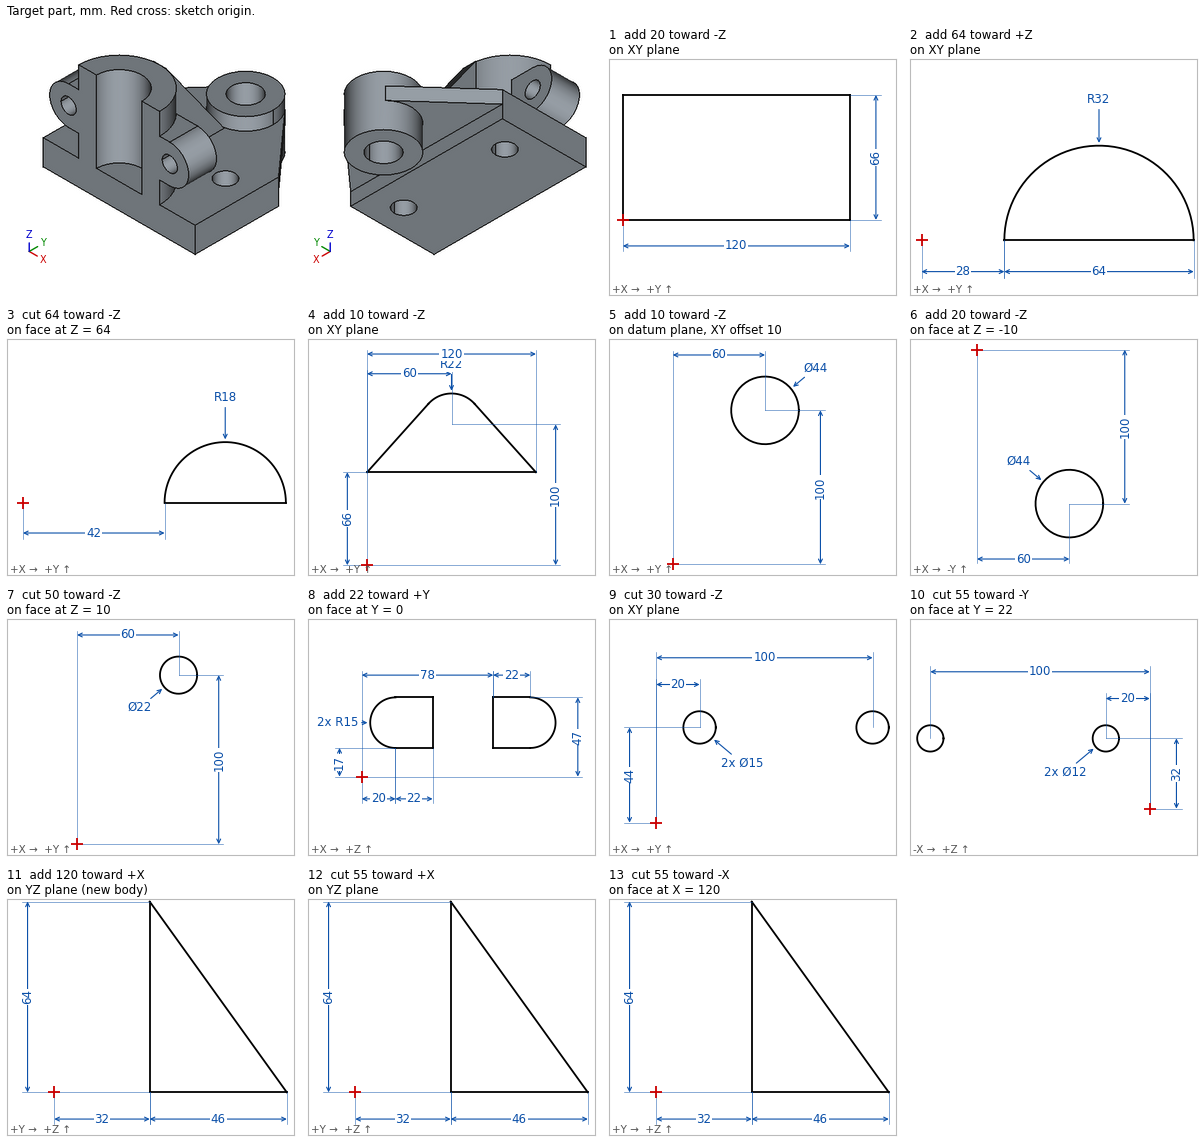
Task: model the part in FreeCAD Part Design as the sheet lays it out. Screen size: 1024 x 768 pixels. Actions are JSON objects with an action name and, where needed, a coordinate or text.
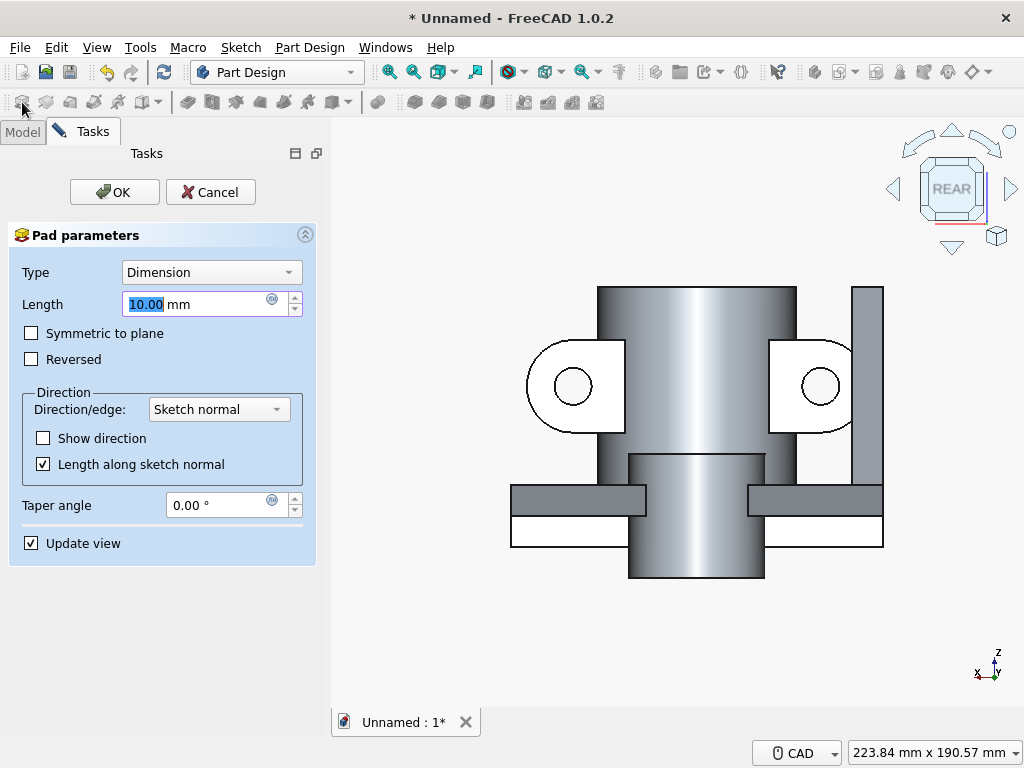
{"action": "type", "text": "120"}
{"action": "key", "text": "Tab"}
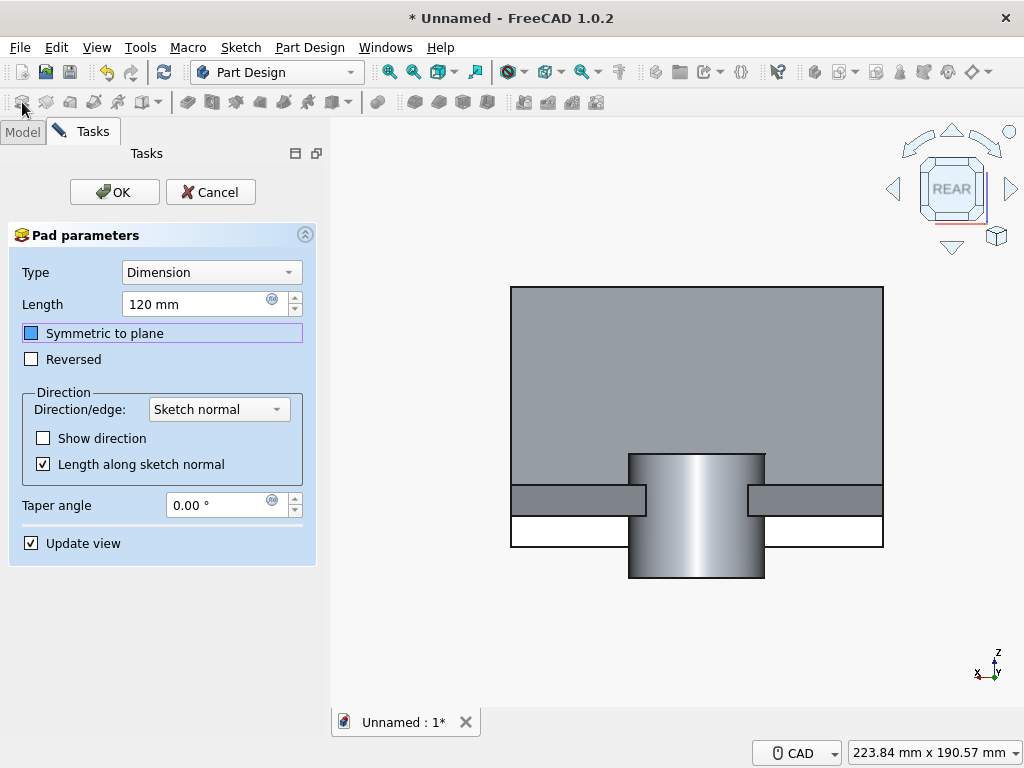
{"action": "left_click", "coordinate": [115, 192]}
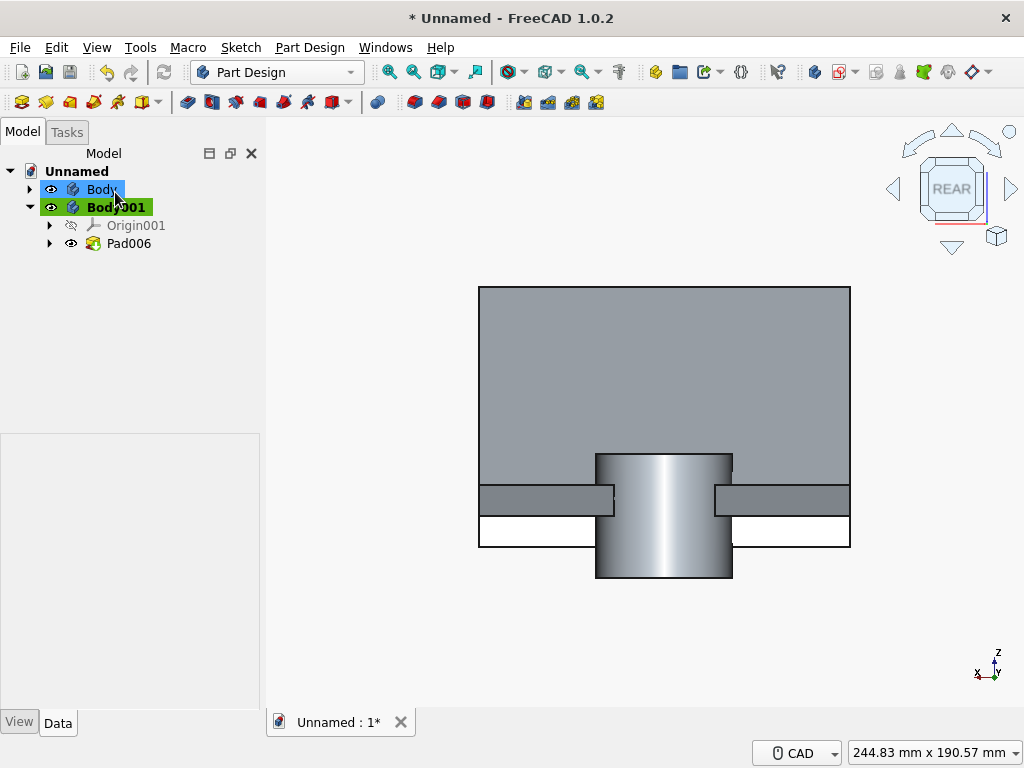
{"action": "left_click", "coordinate": [840, 72]}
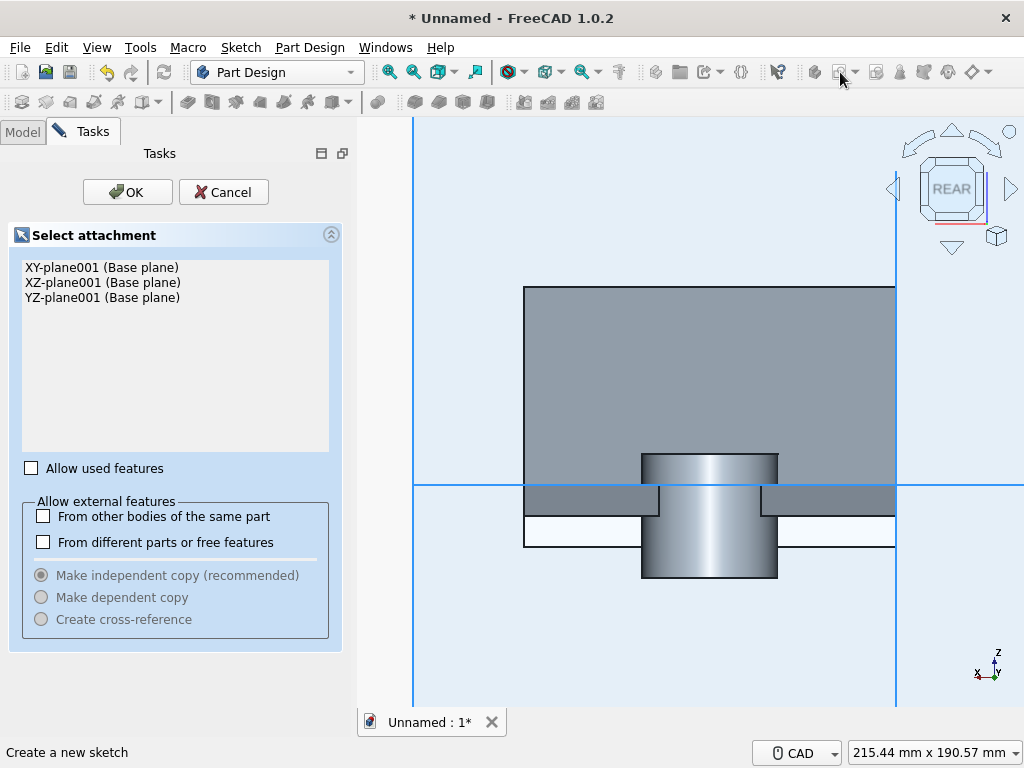
{"action": "left_click", "coordinate": [82, 298]}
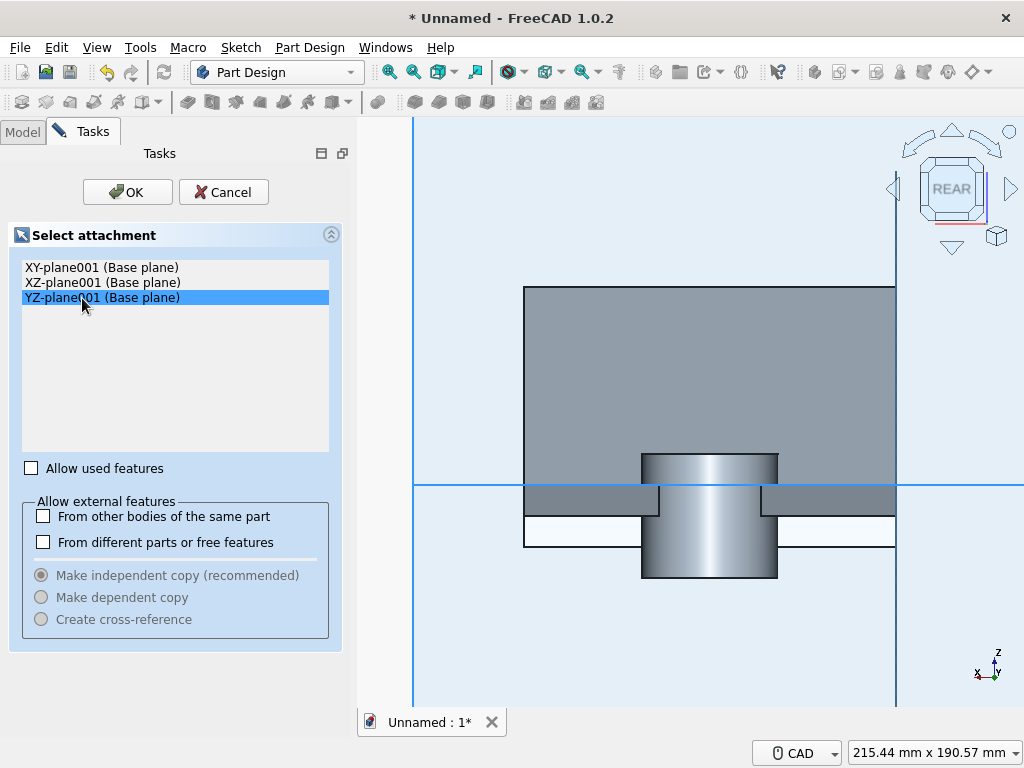
{"action": "left_click", "coordinate": [128, 192]}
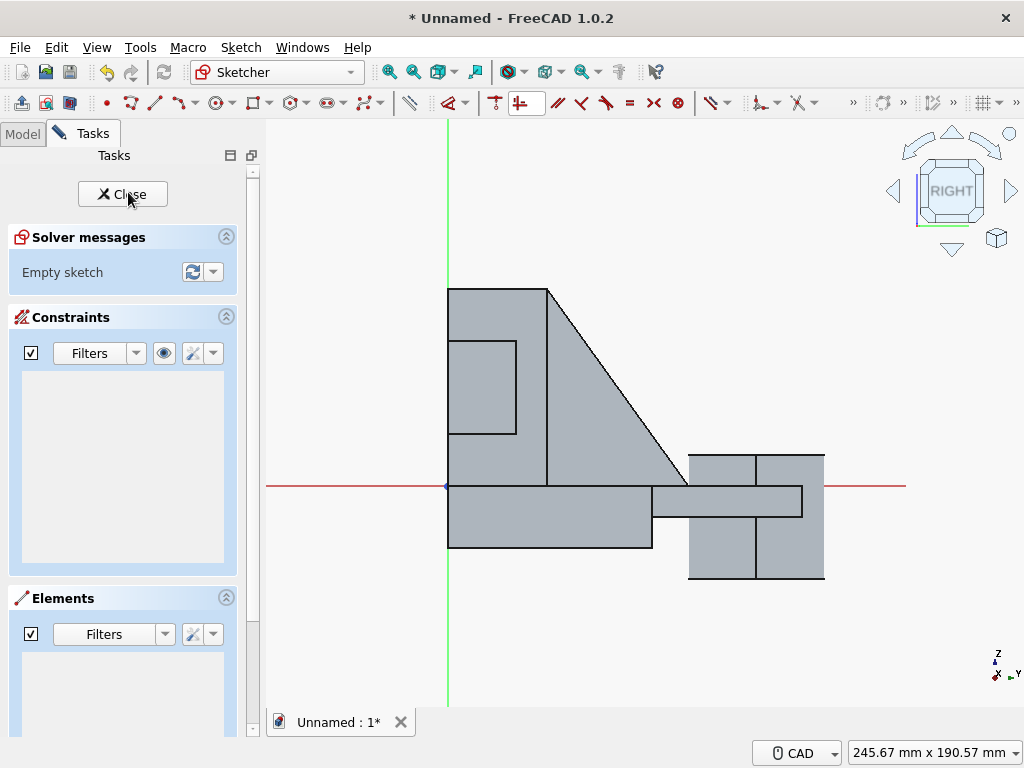
{"action": "left_click", "coordinate": [70, 104]}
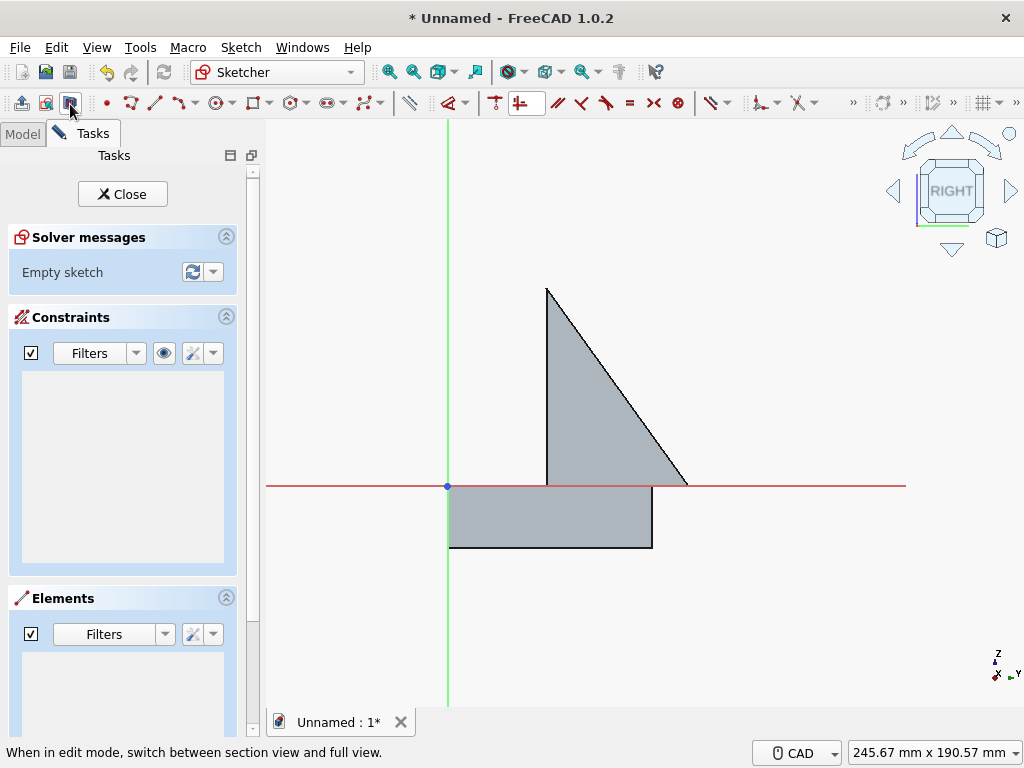
{"action": "scroll", "coordinate": [558, 356], "scroll_direction": "up", "scroll_amount": 3}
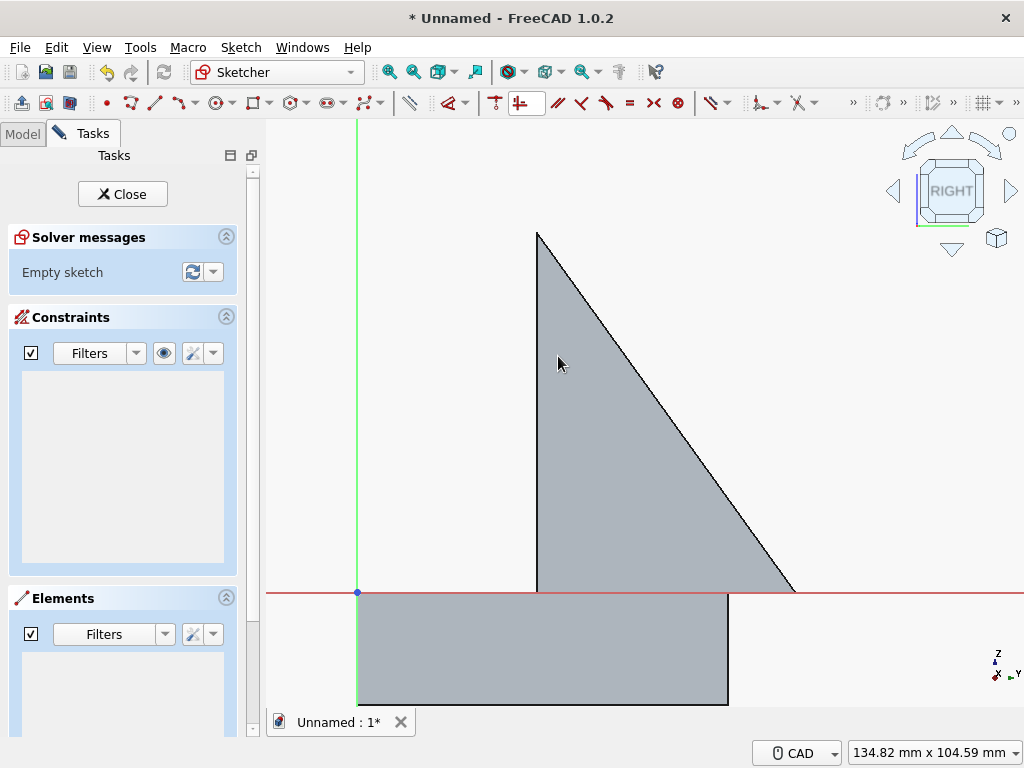
{"action": "left_click", "coordinate": [132, 104]}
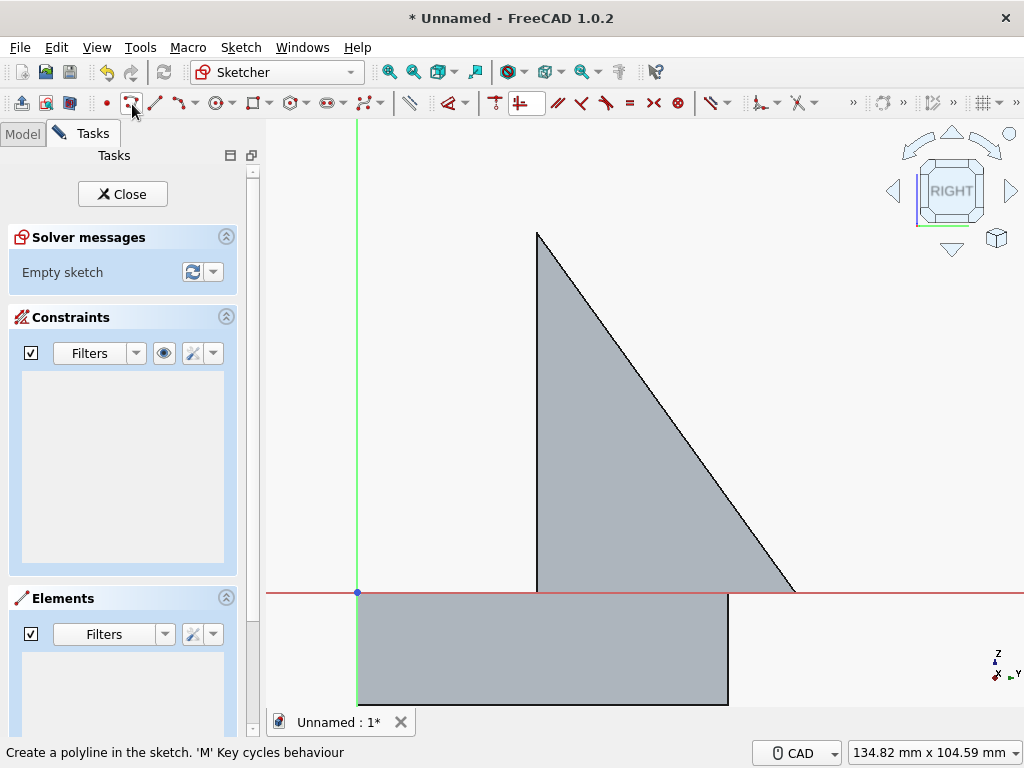
{"action": "left_click", "coordinate": [537, 593]}
{"action": "left_click", "coordinate": [537, 233]}
{"action": "left_click", "coordinate": [796, 584]}
{"action": "left_click", "coordinate": [537, 593]}
{"action": "key", "text": "Escape"}
{"action": "key", "text": "Escape"}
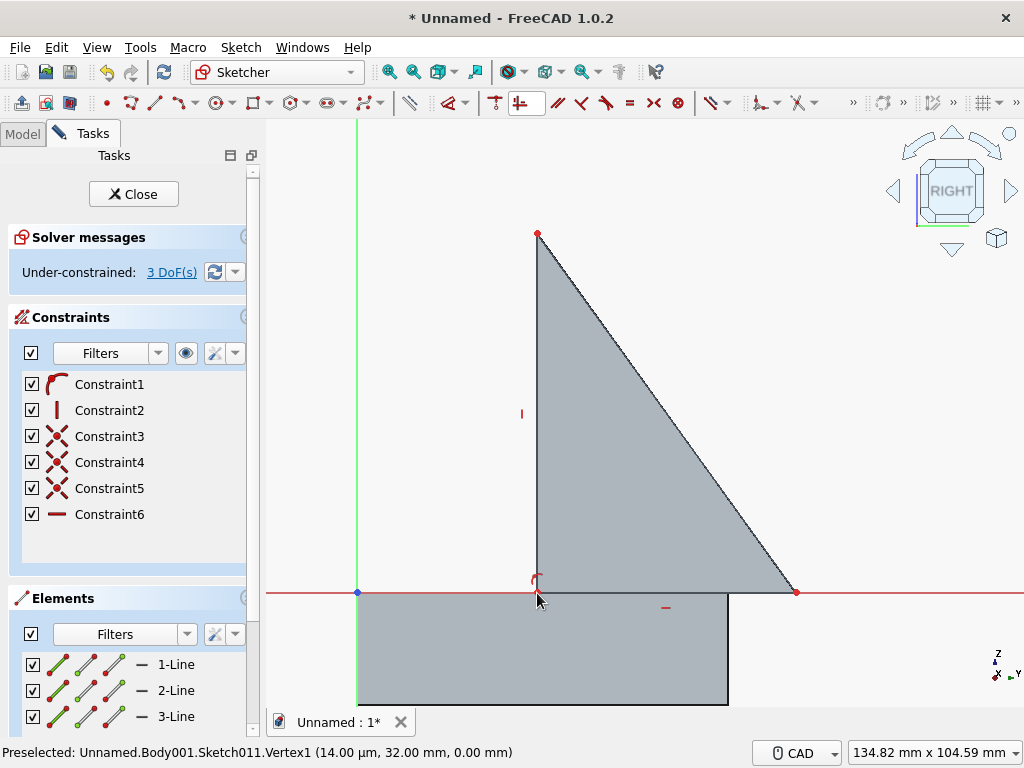
{"action": "left_click", "coordinate": [448, 104]}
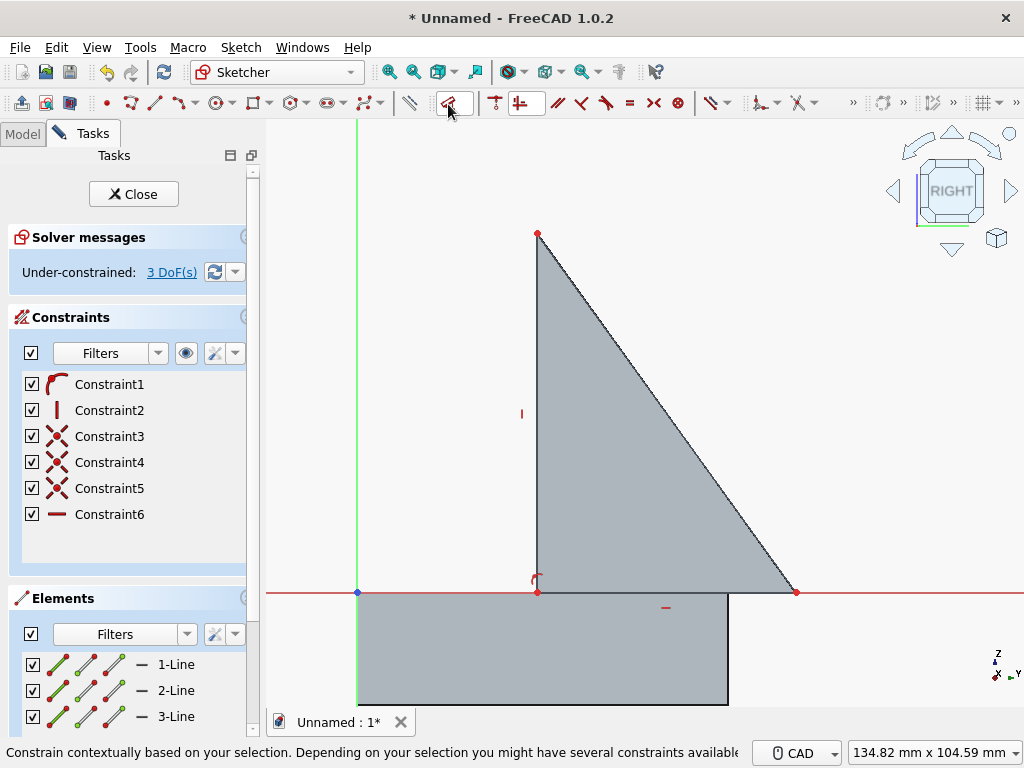
{"action": "left_click", "coordinate": [537, 485]}
{"action": "left_click", "coordinate": [503, 413]}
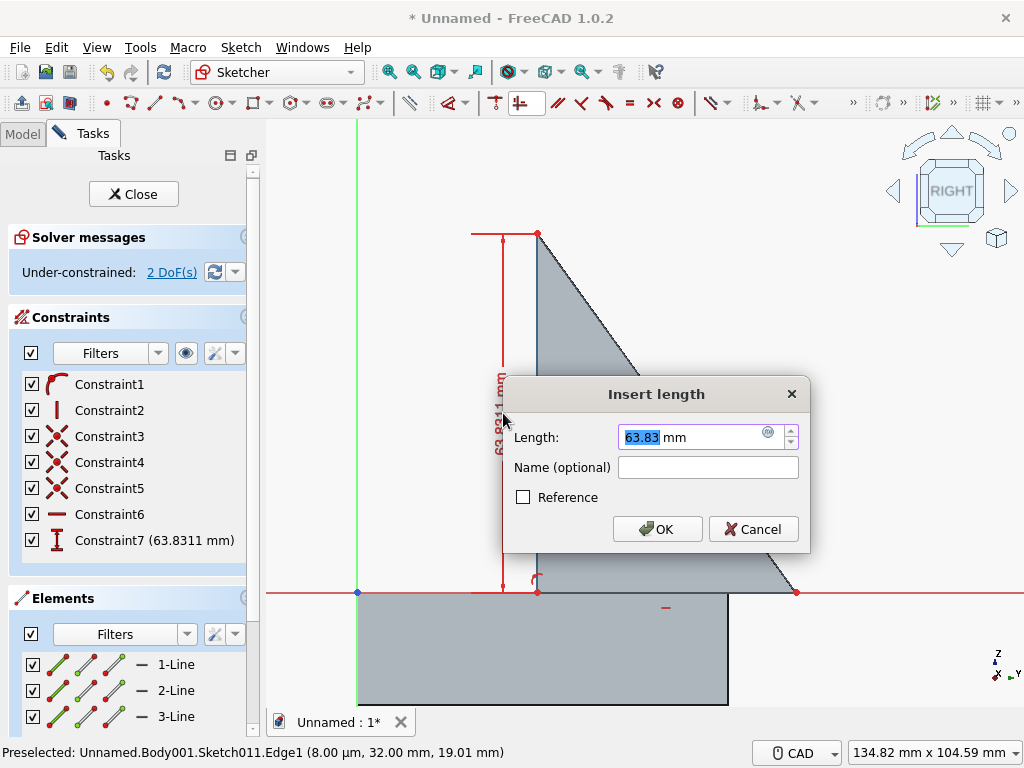
{"action": "type", "text": "64"}
{"action": "key", "text": "Return"}